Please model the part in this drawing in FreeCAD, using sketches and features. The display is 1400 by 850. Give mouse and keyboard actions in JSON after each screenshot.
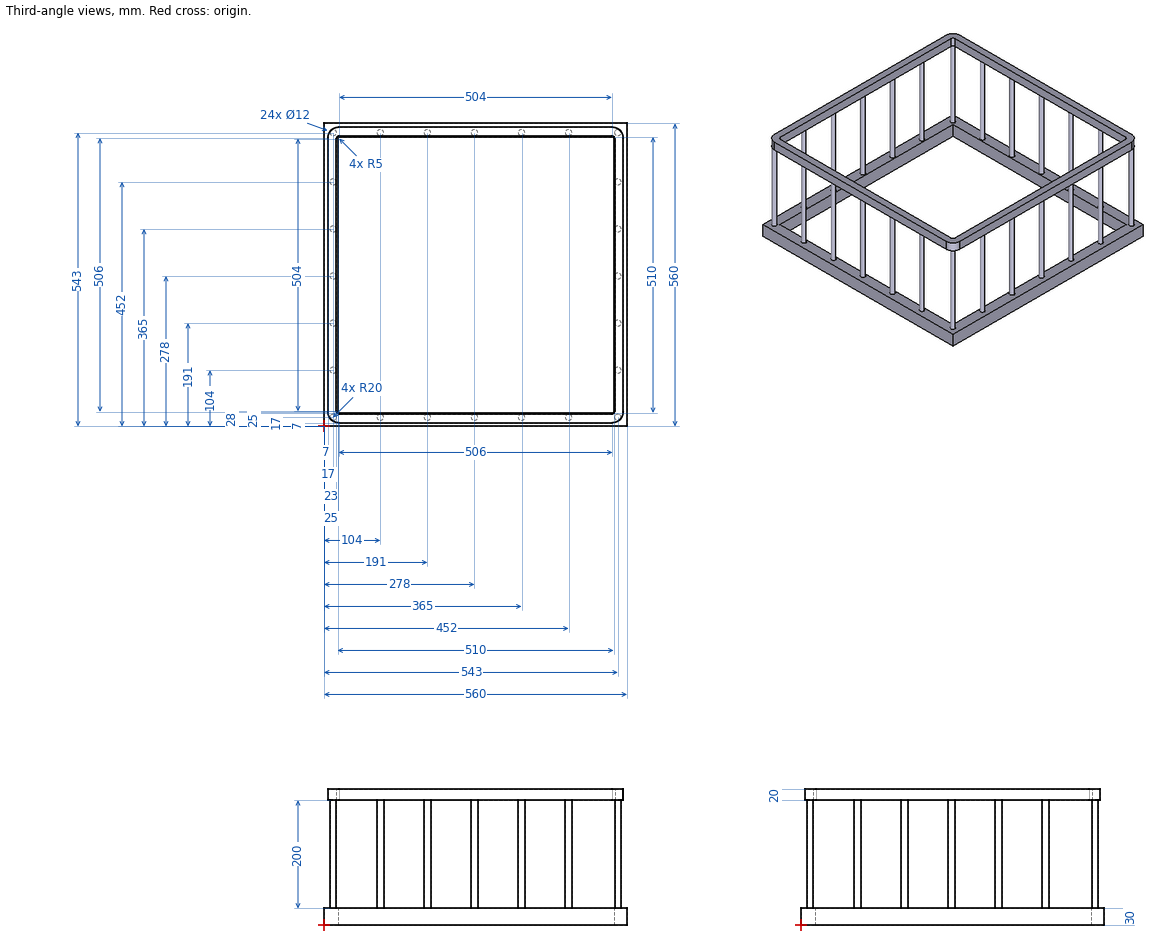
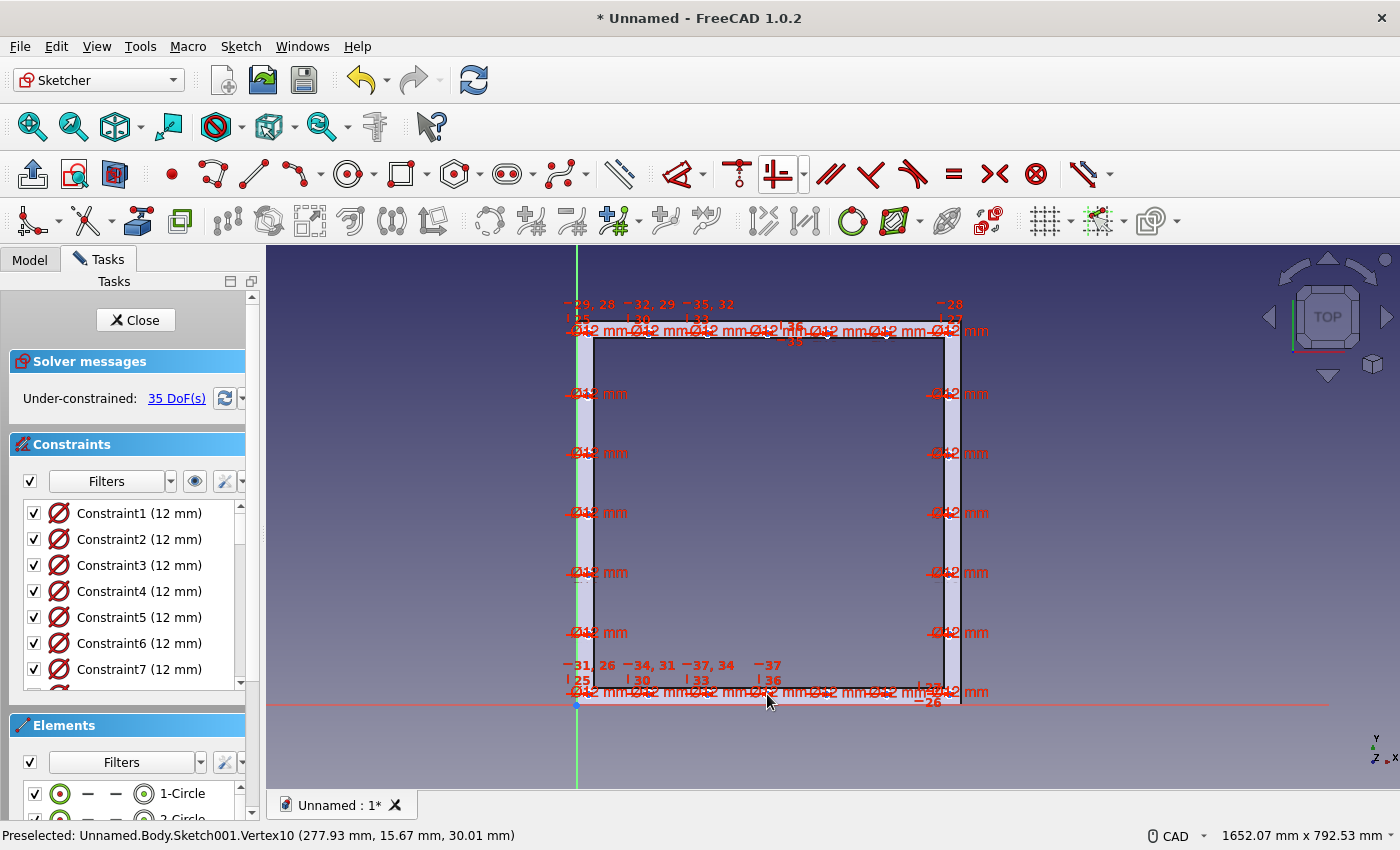
{"action": "left_click", "coordinate": [767, 333]}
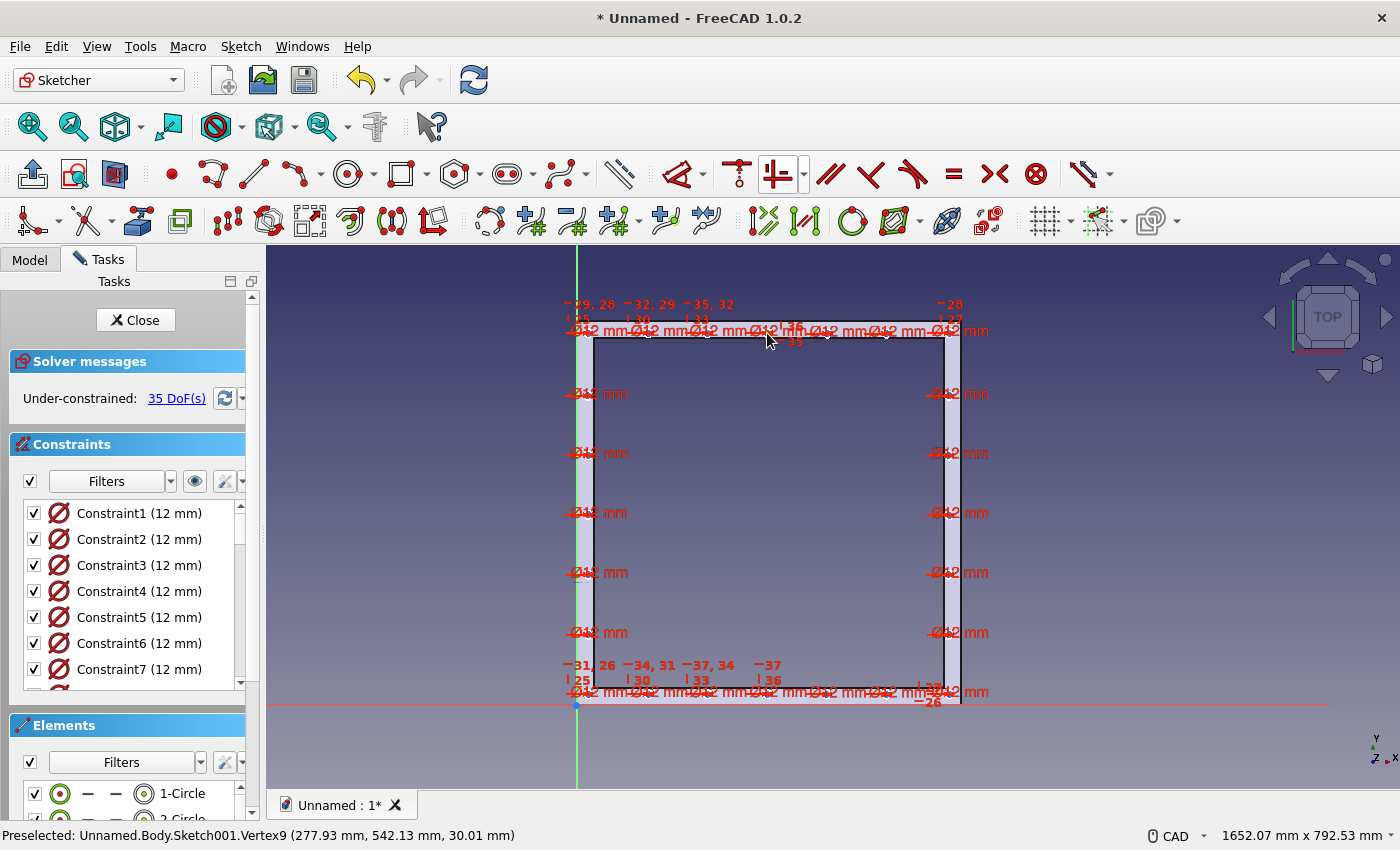
{"action": "left_click", "coordinate": [827, 334]}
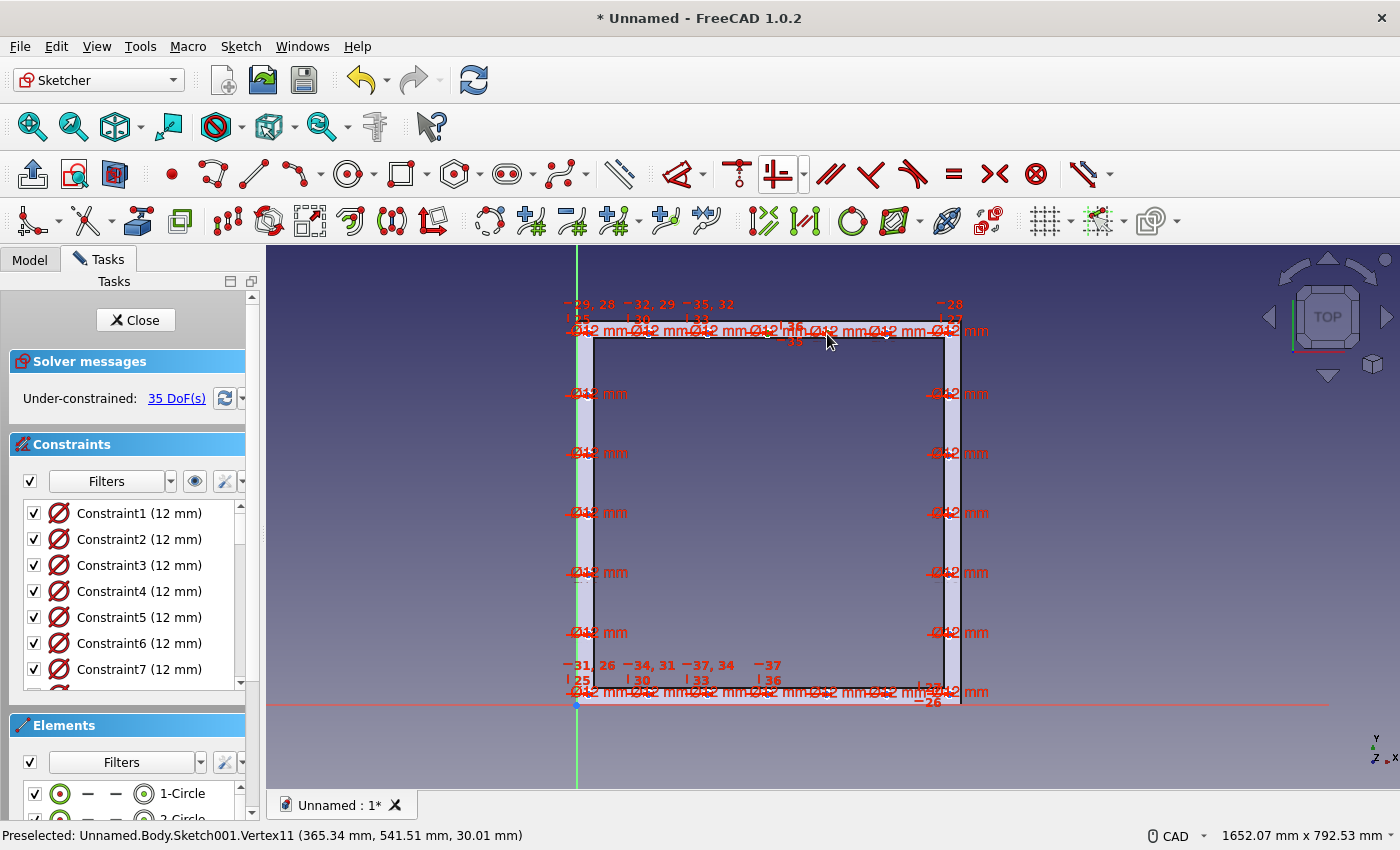
{"action": "key", "text": "h"}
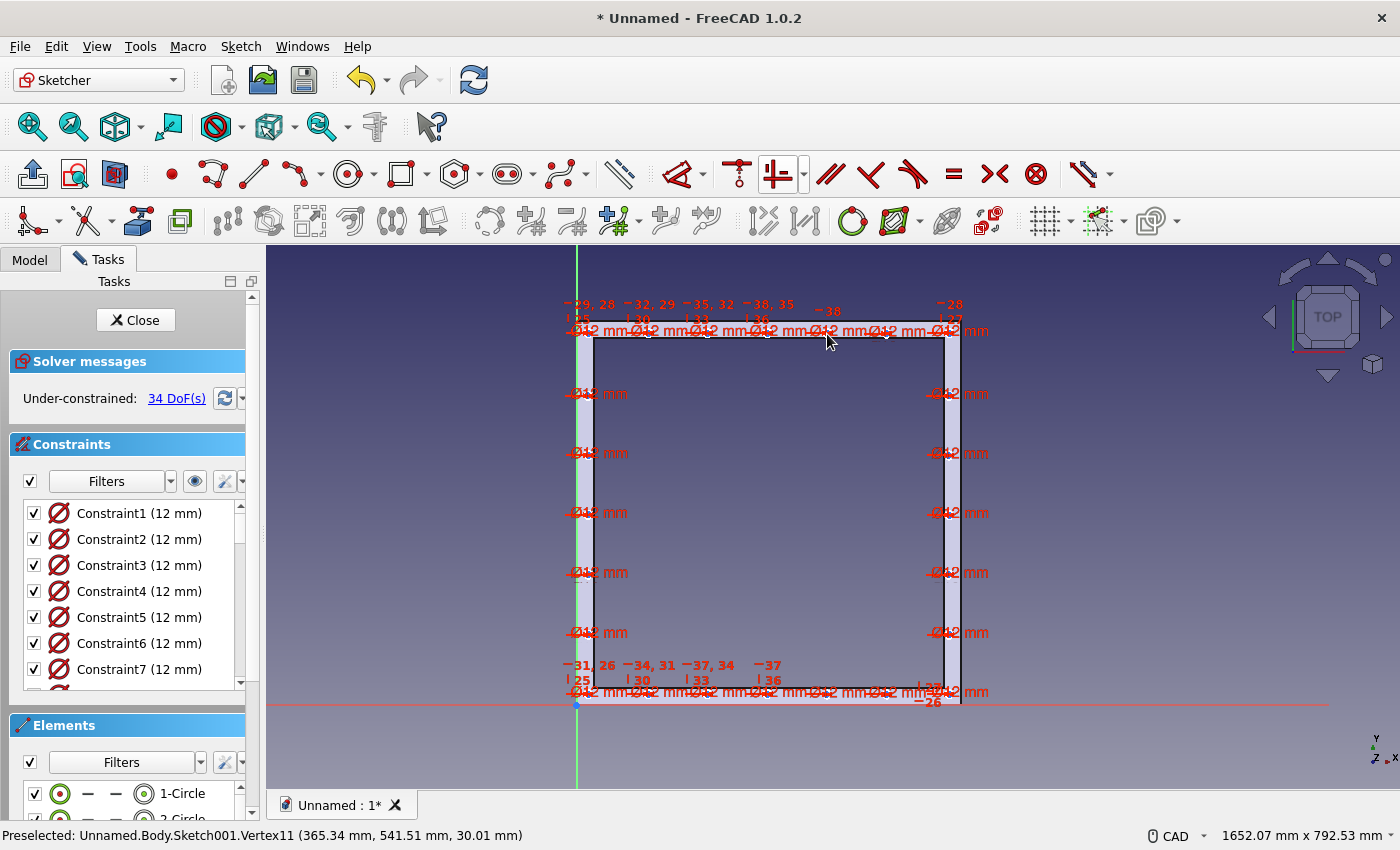
{"action": "left_click", "coordinate": [827, 333]}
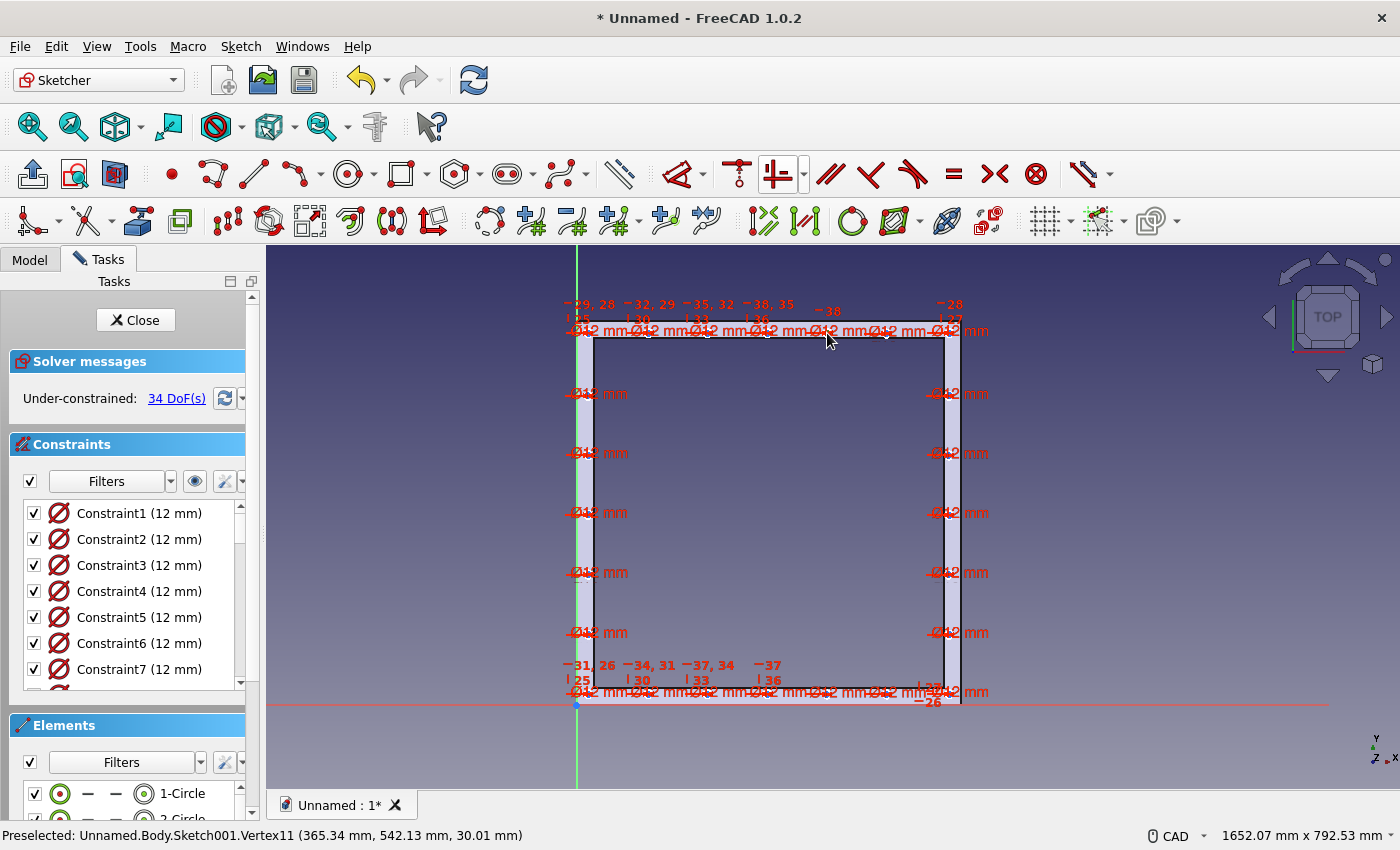
{"action": "left_click", "coordinate": [827, 694]}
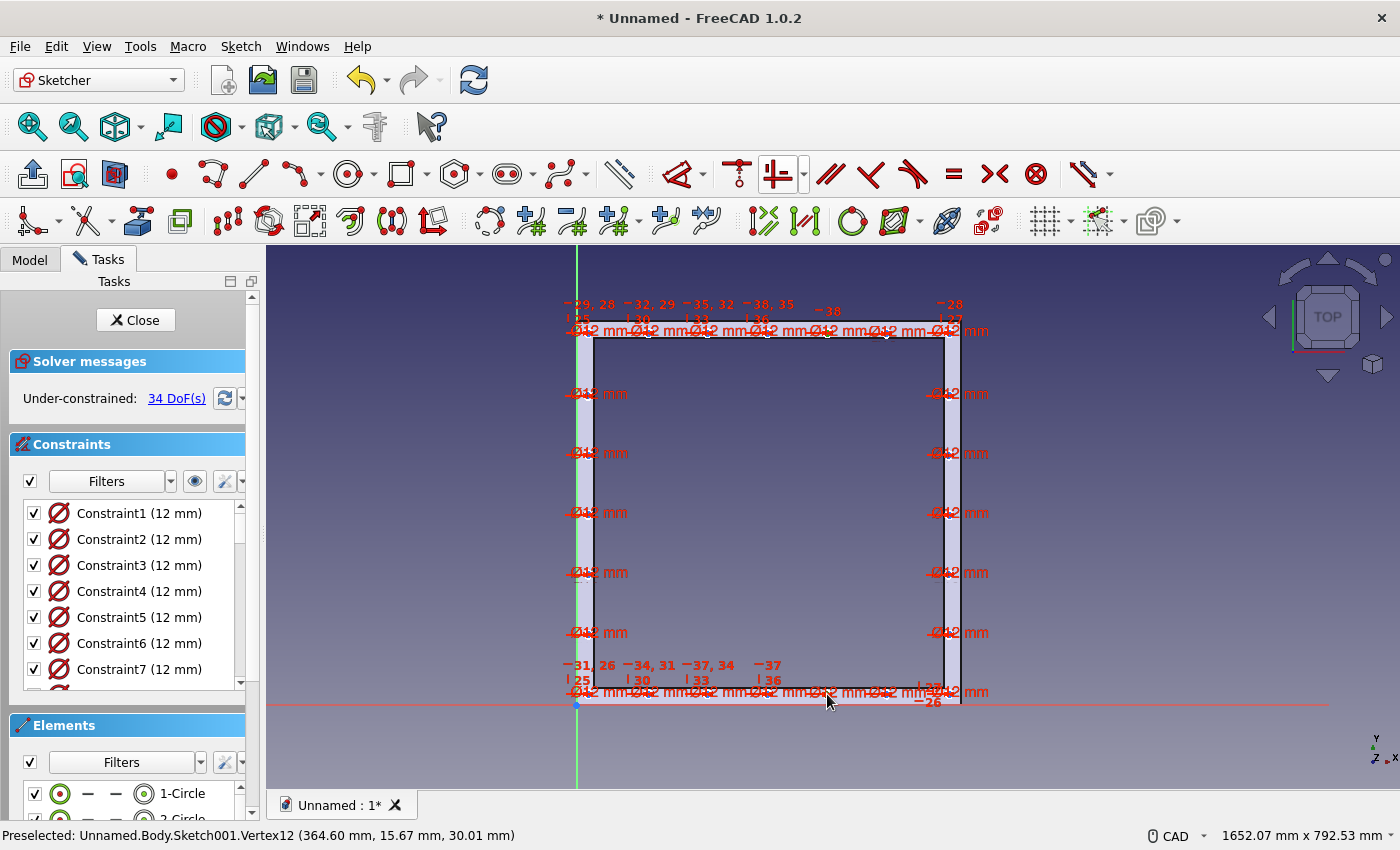
{"action": "key", "text": "v"}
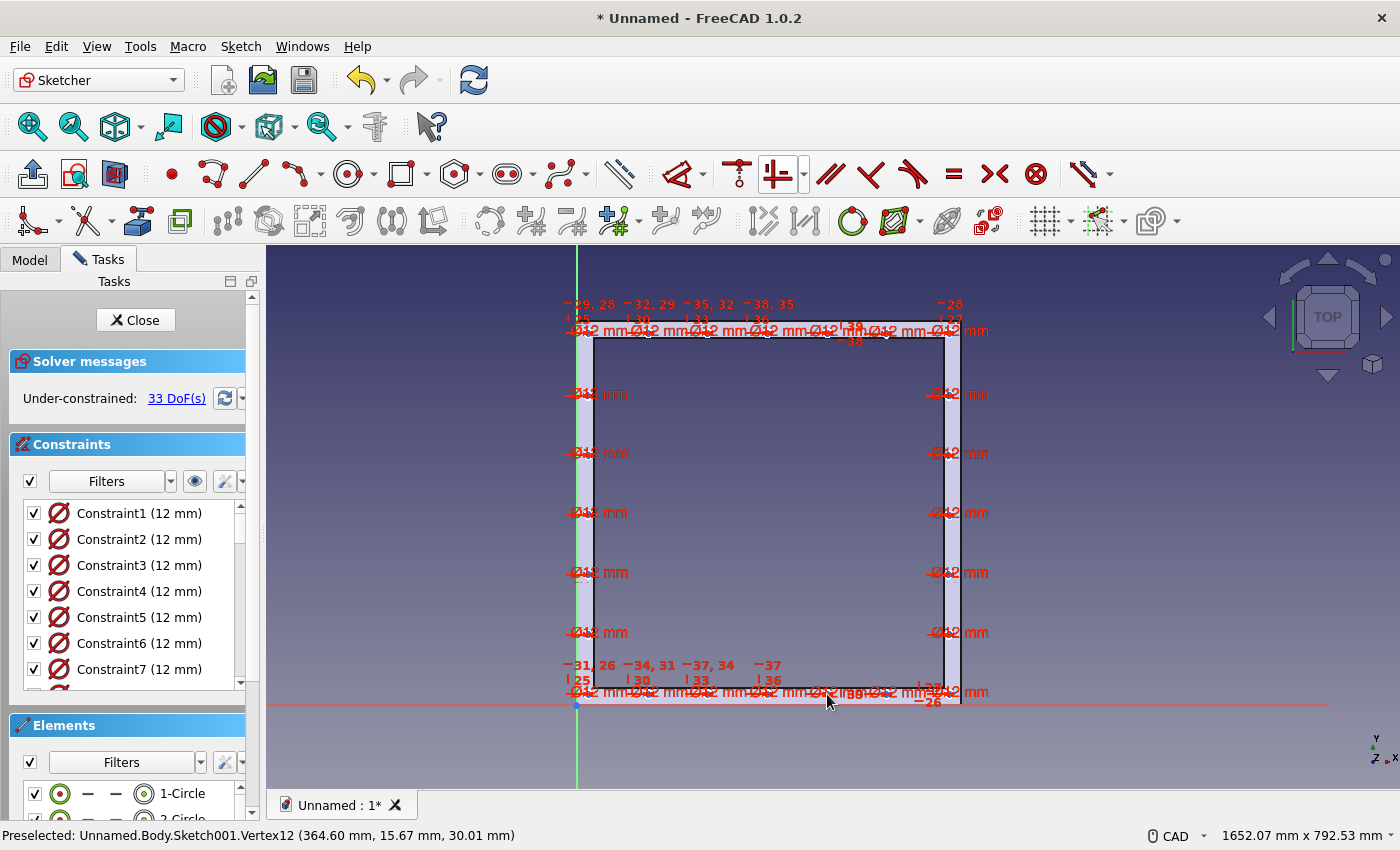
{"action": "left_click", "coordinate": [767, 694]}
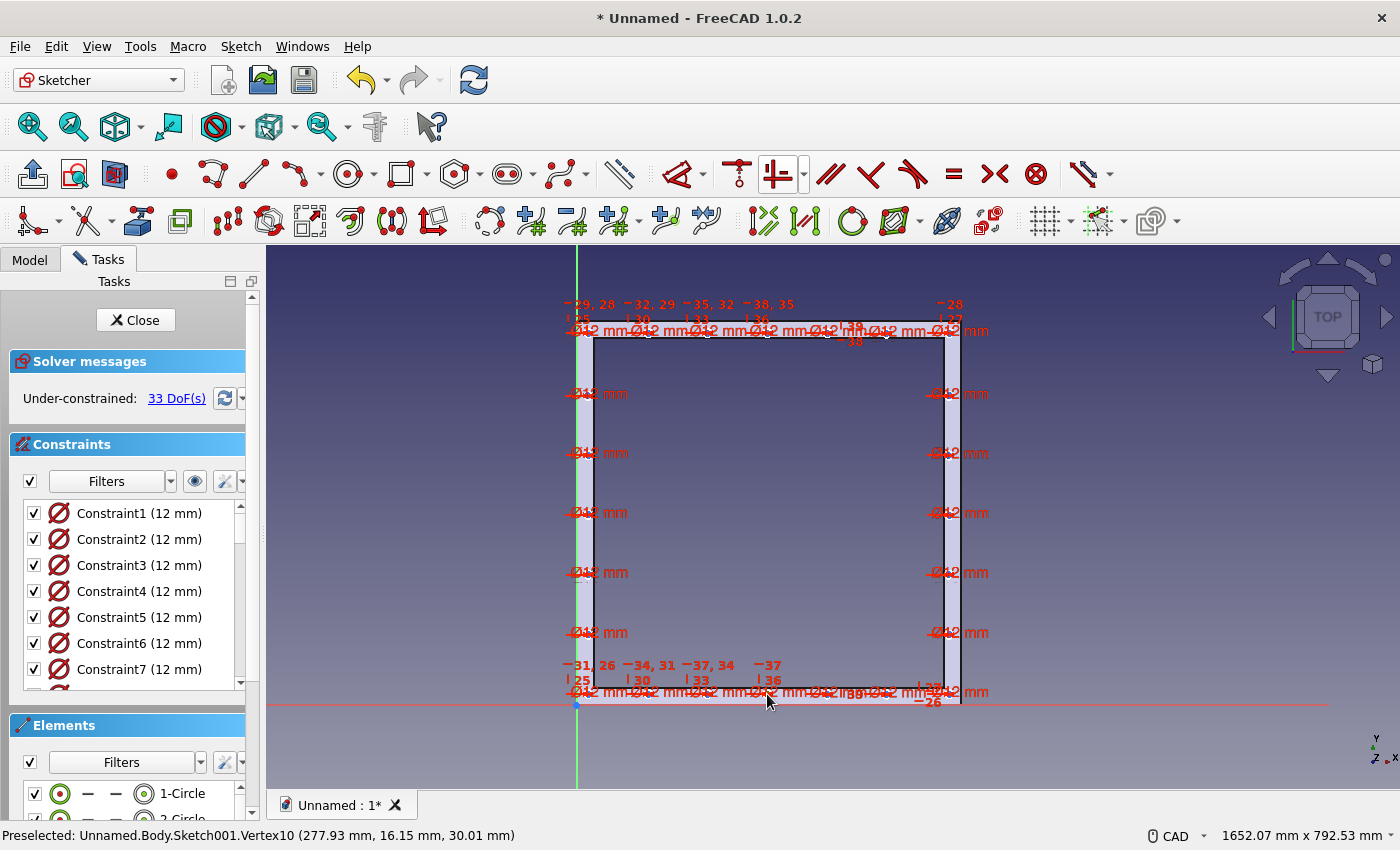
{"action": "left_click", "coordinate": [827, 694]}